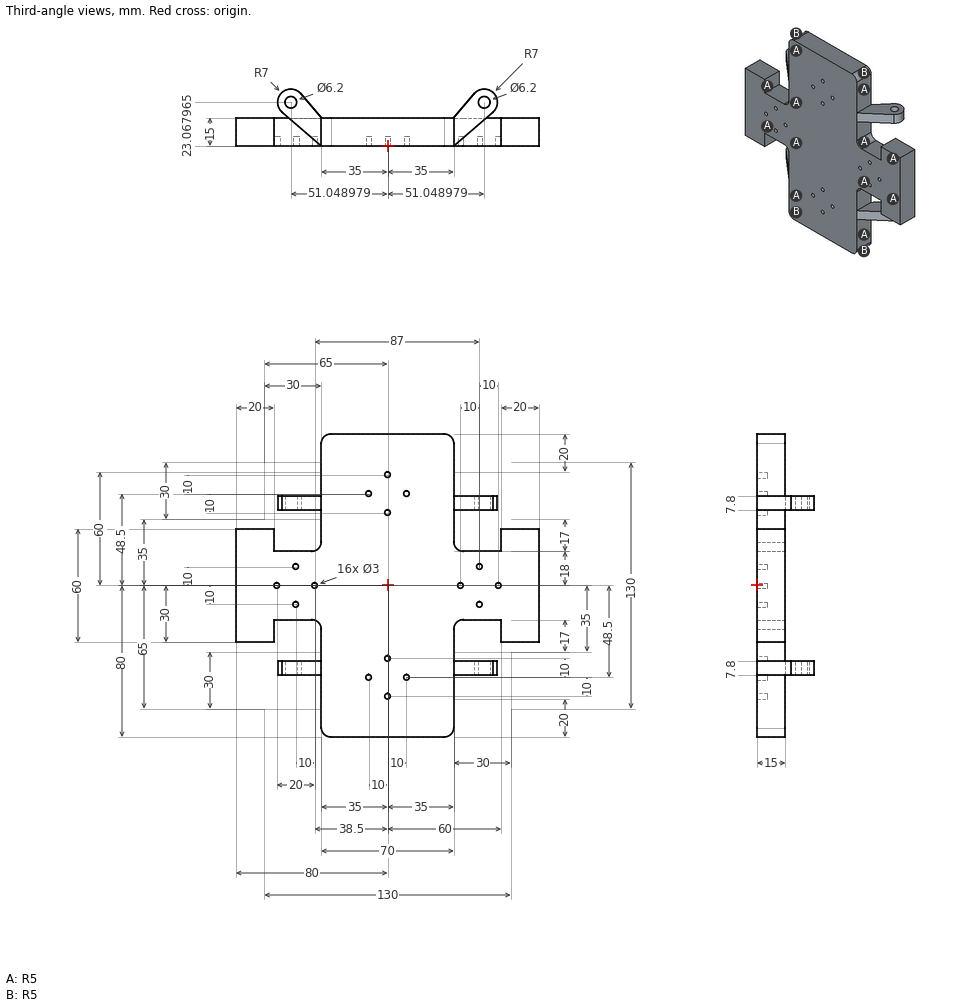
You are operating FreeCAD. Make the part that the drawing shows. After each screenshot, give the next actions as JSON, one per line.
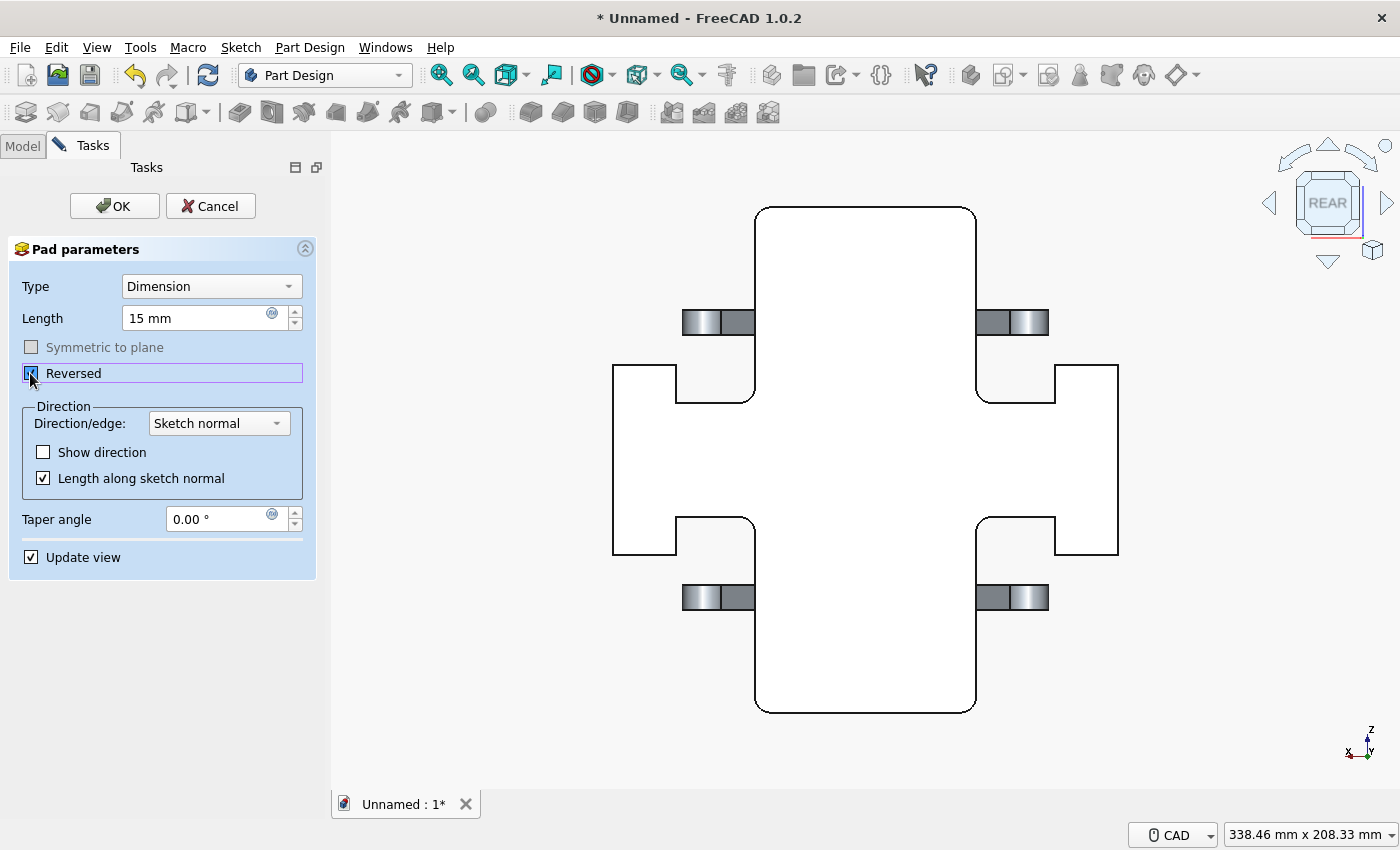
{"action": "left_click", "coordinate": [115, 206]}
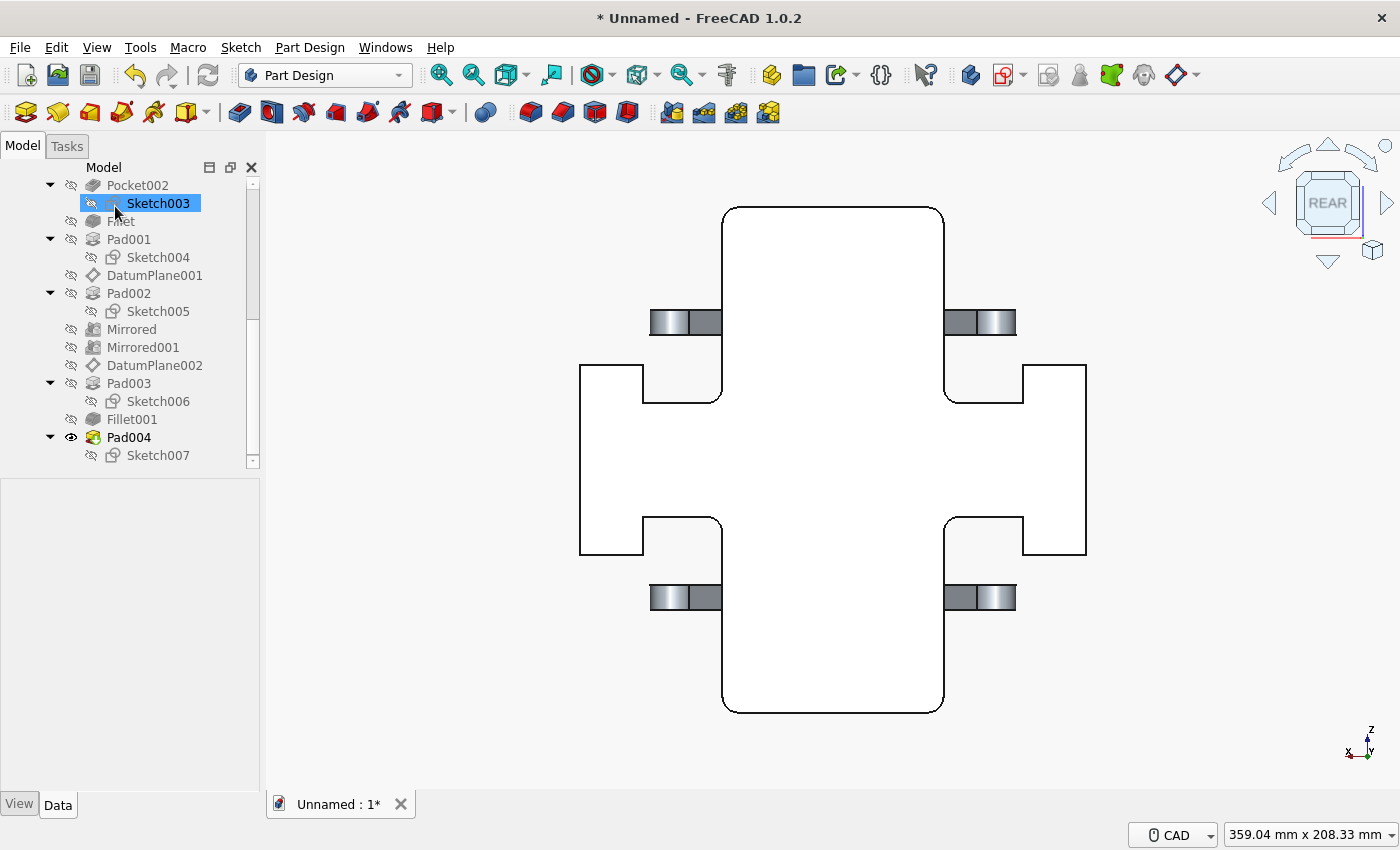
{"action": "key", "text": "0"}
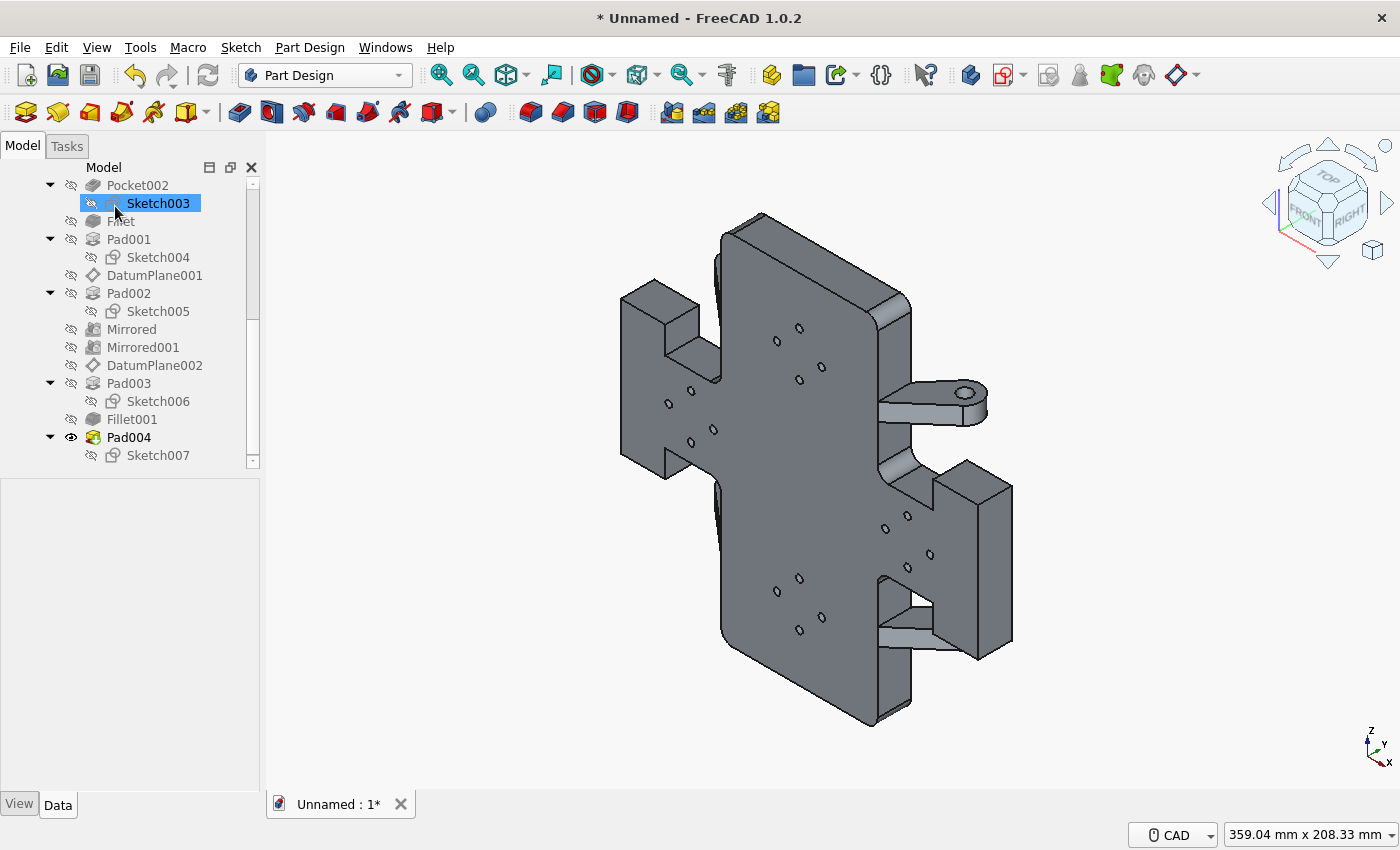
{"action": "key", "text": "v f"}